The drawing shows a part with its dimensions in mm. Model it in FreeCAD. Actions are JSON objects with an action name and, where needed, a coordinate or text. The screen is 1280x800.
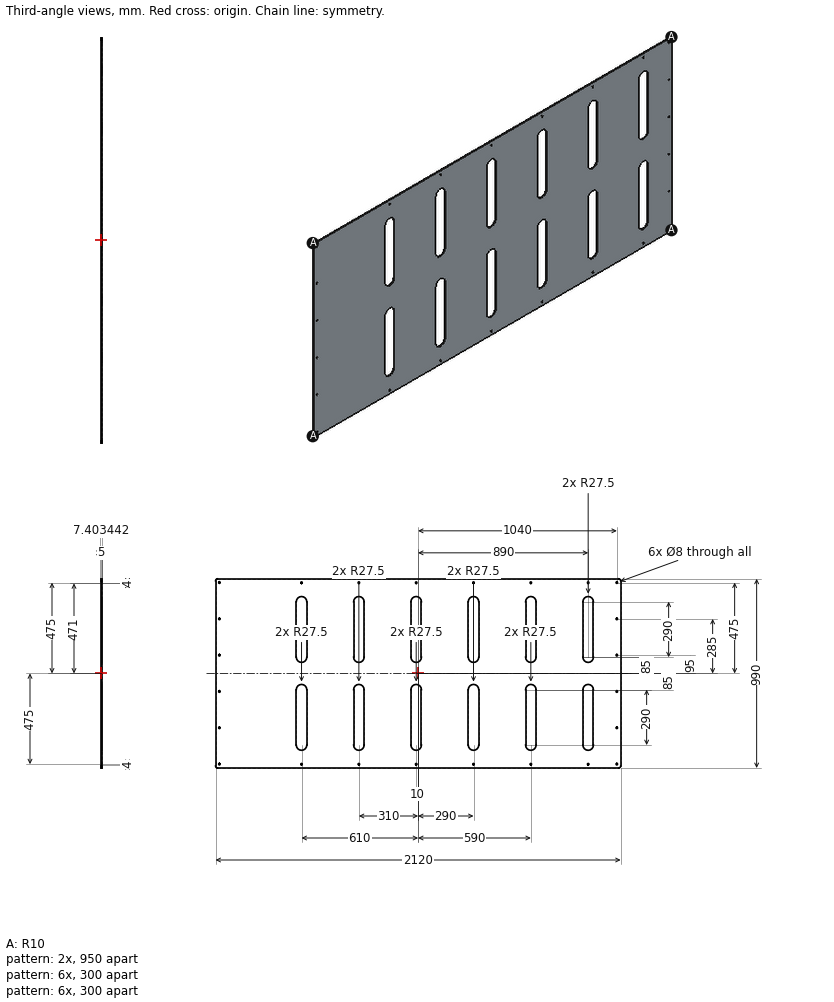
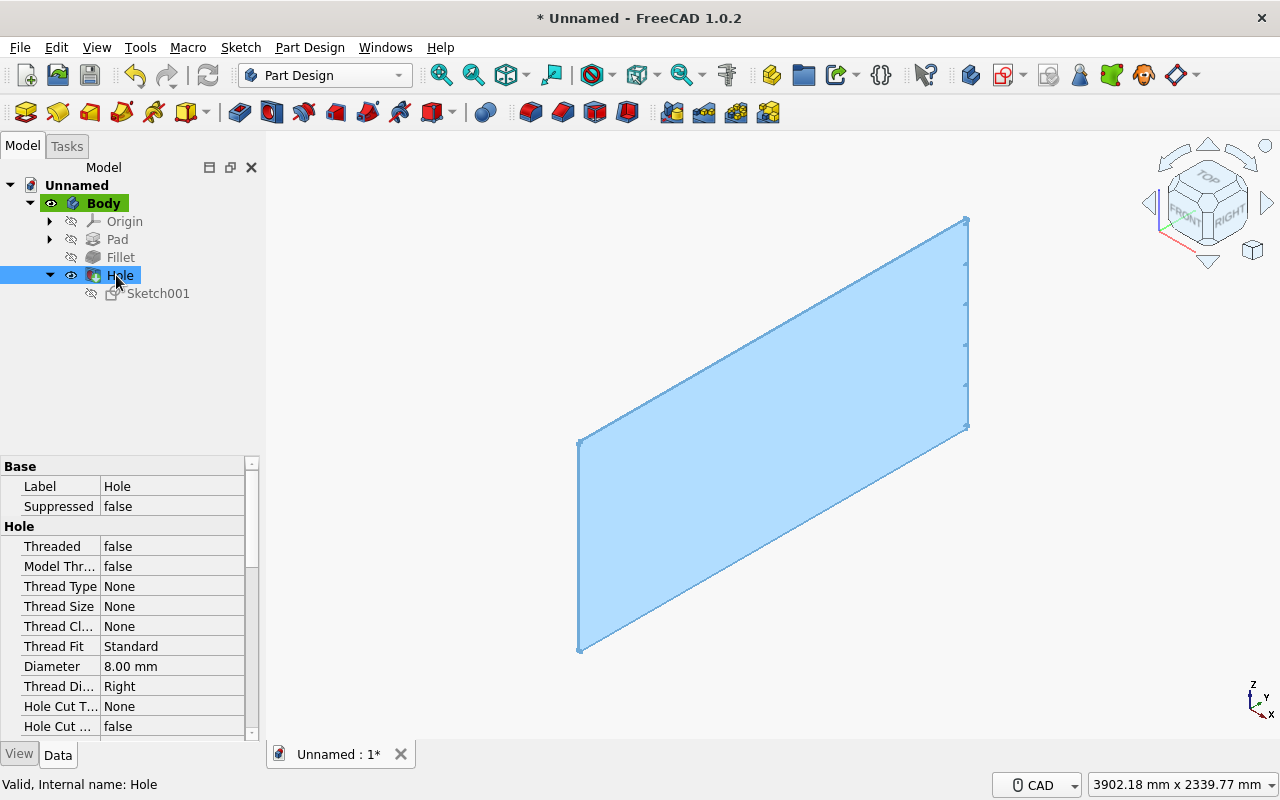
{"action": "left_click", "coordinate": [672, 112]}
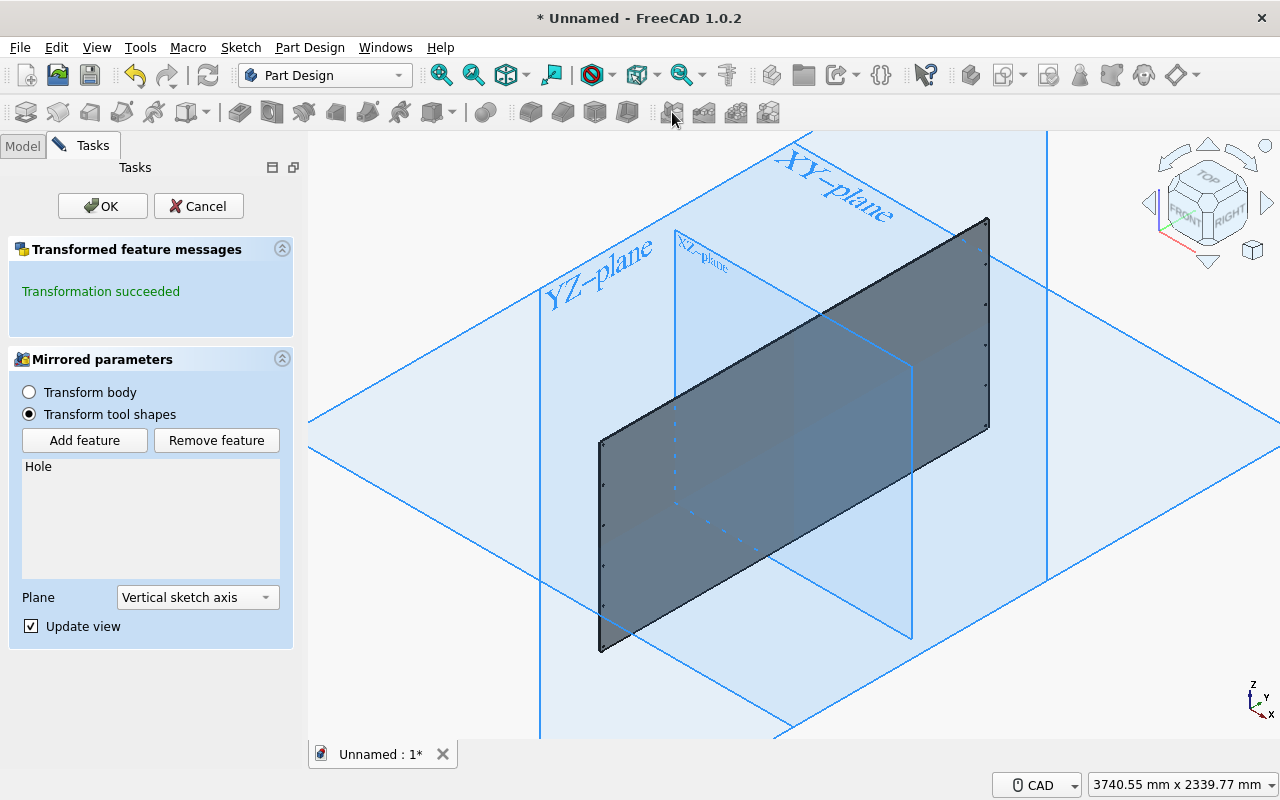
{"action": "left_click", "coordinate": [198, 598]}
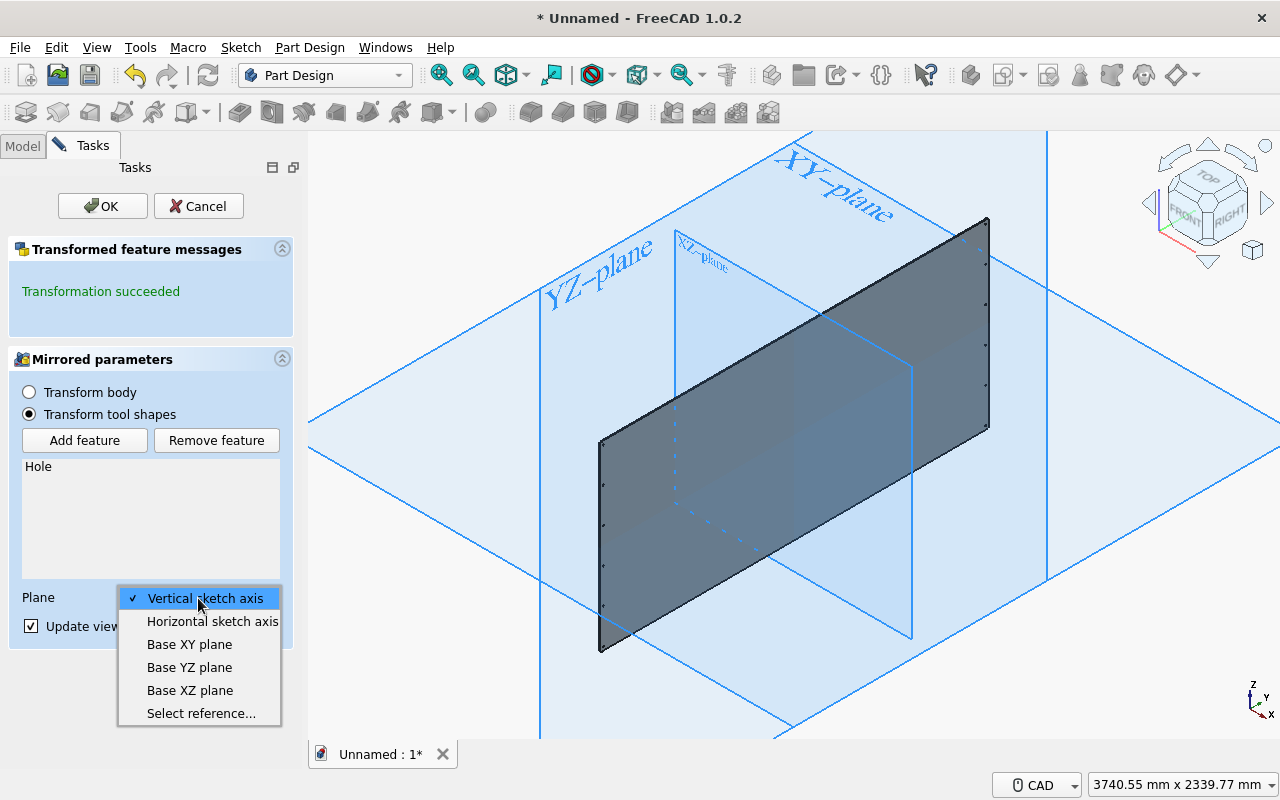
{"action": "left_click", "coordinate": [198, 690]}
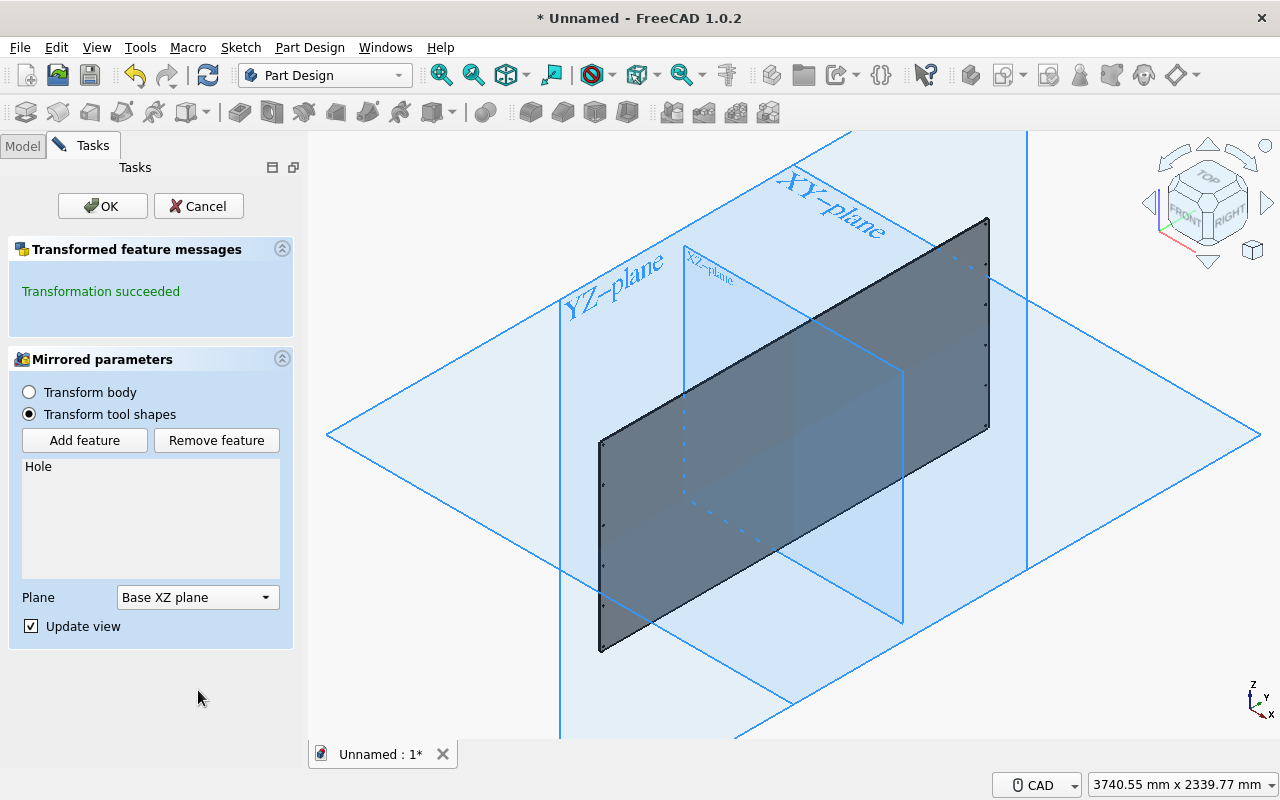
{"action": "left_click", "coordinate": [103, 206]}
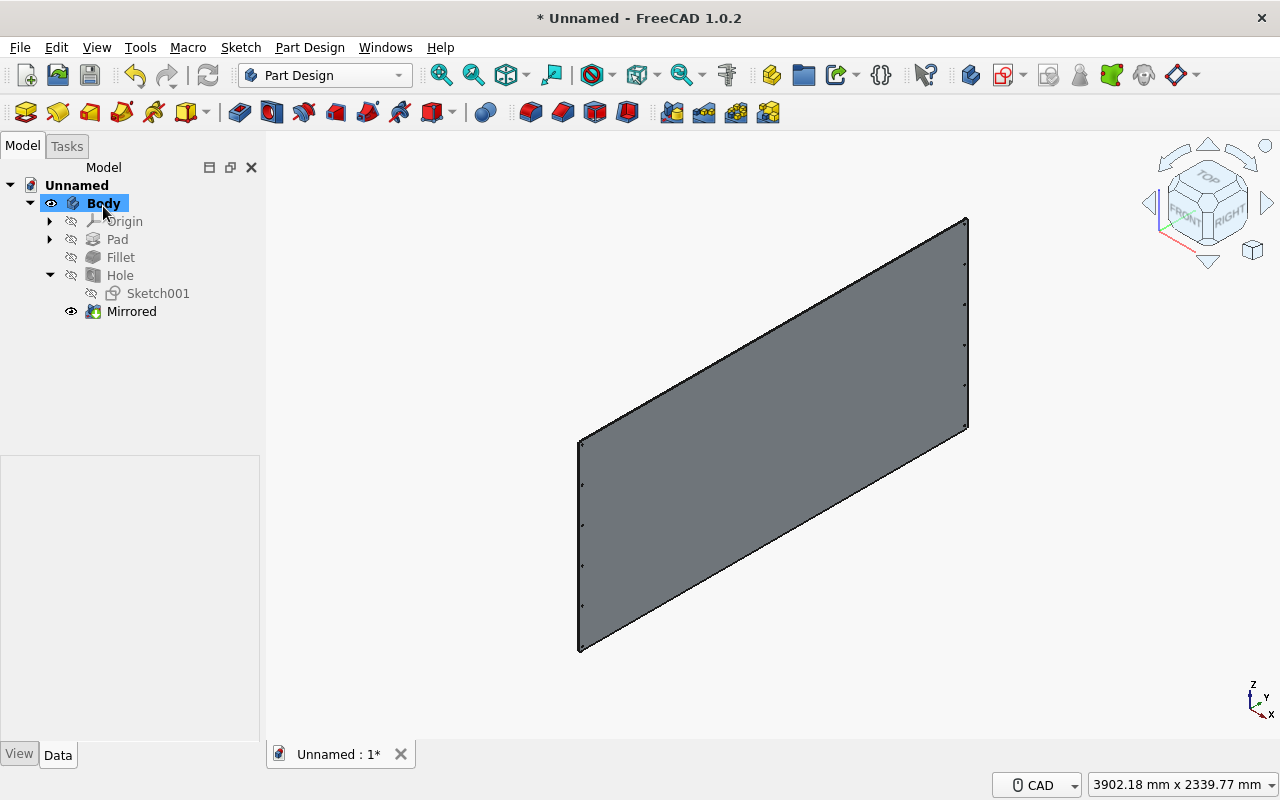
{"action": "left_click", "coordinate": [50, 221]}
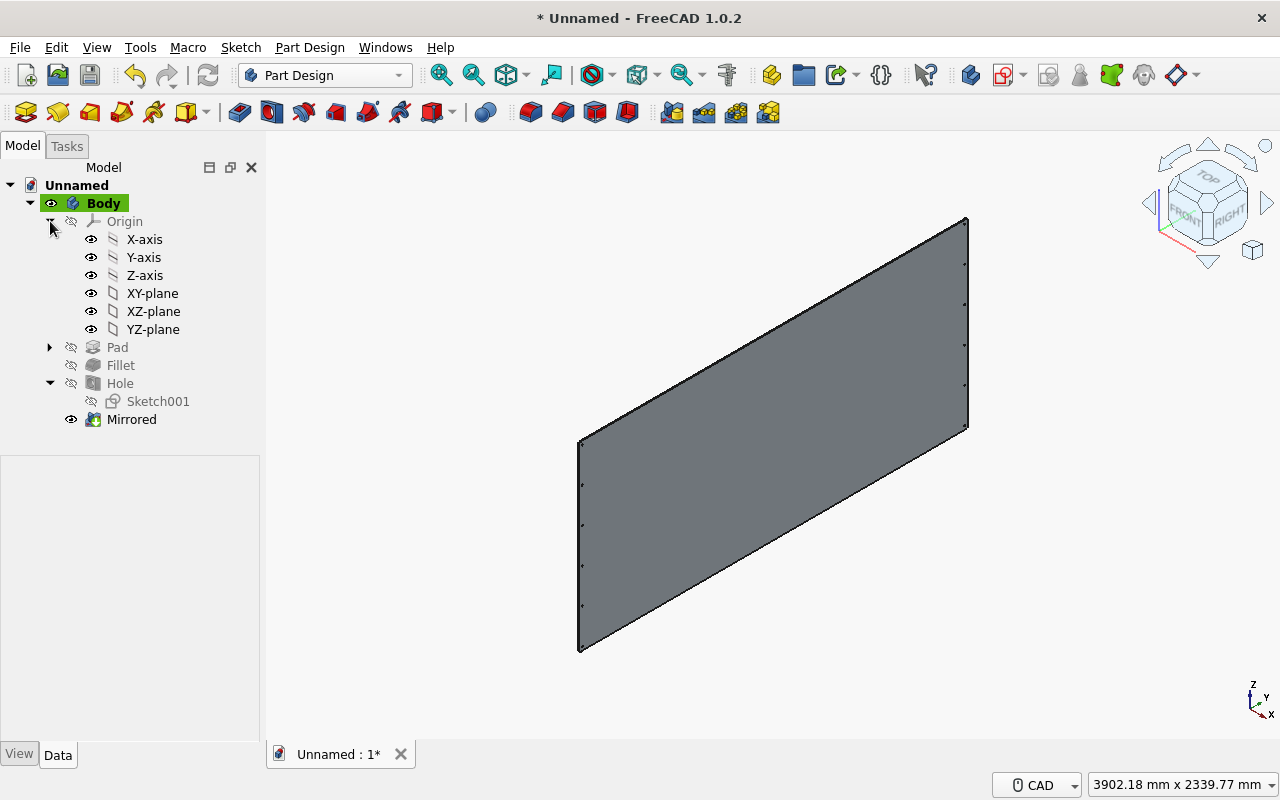
{"action": "left_click", "coordinate": [136, 311]}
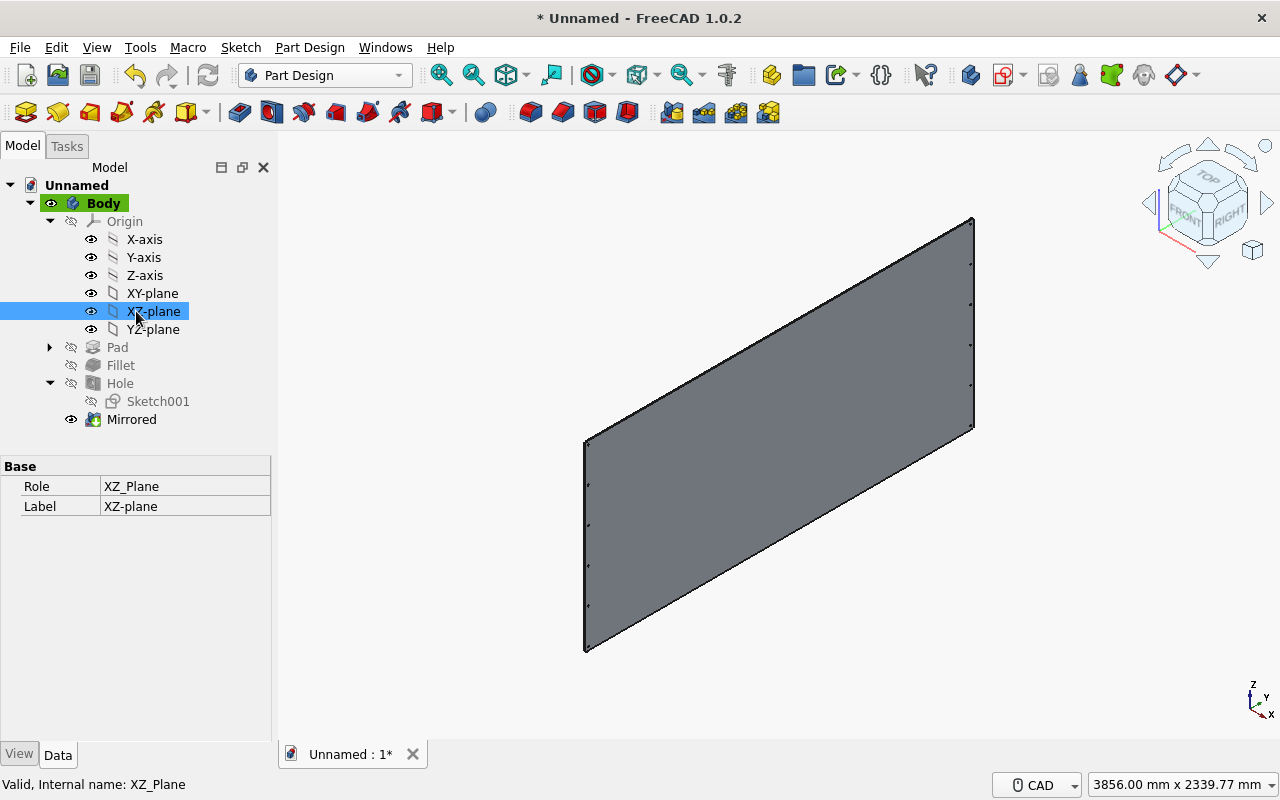
{"action": "left_click", "coordinate": [1176, 76]}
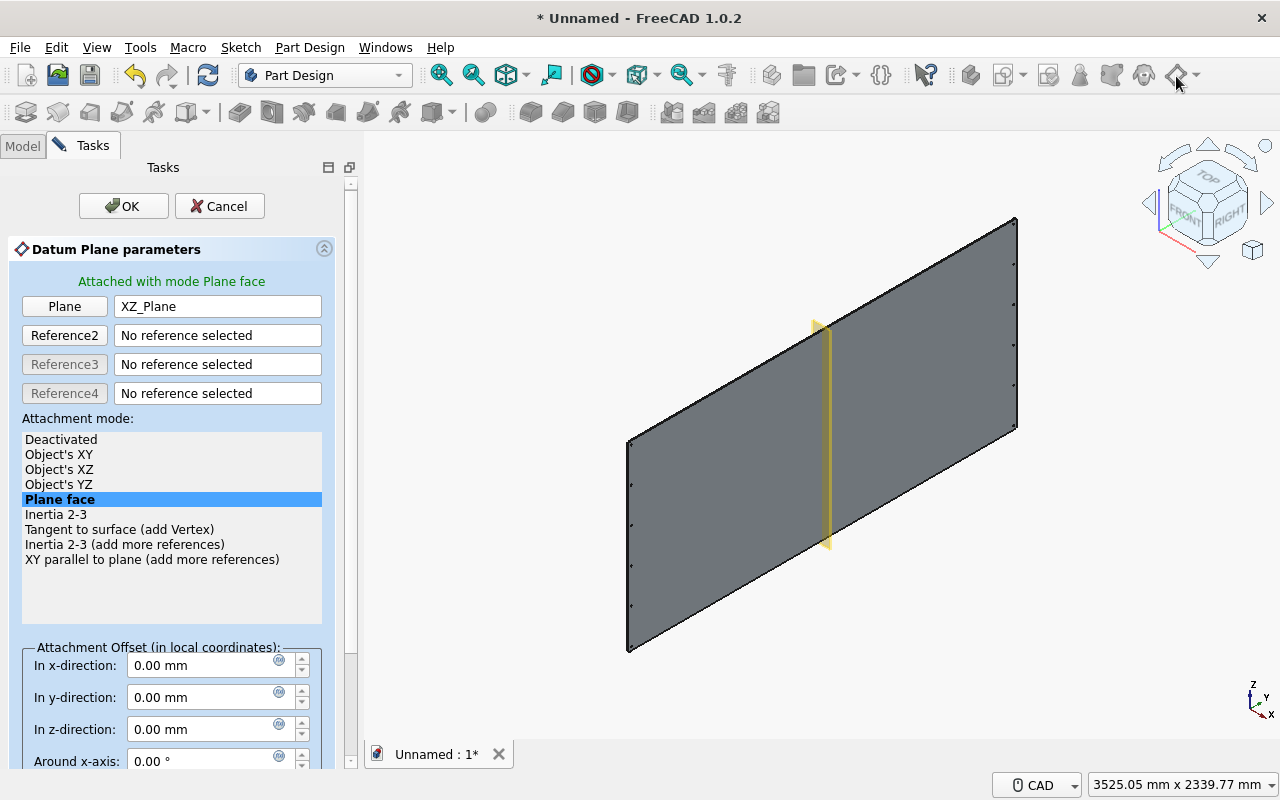
{"action": "triple_click", "coordinate": [210, 729]}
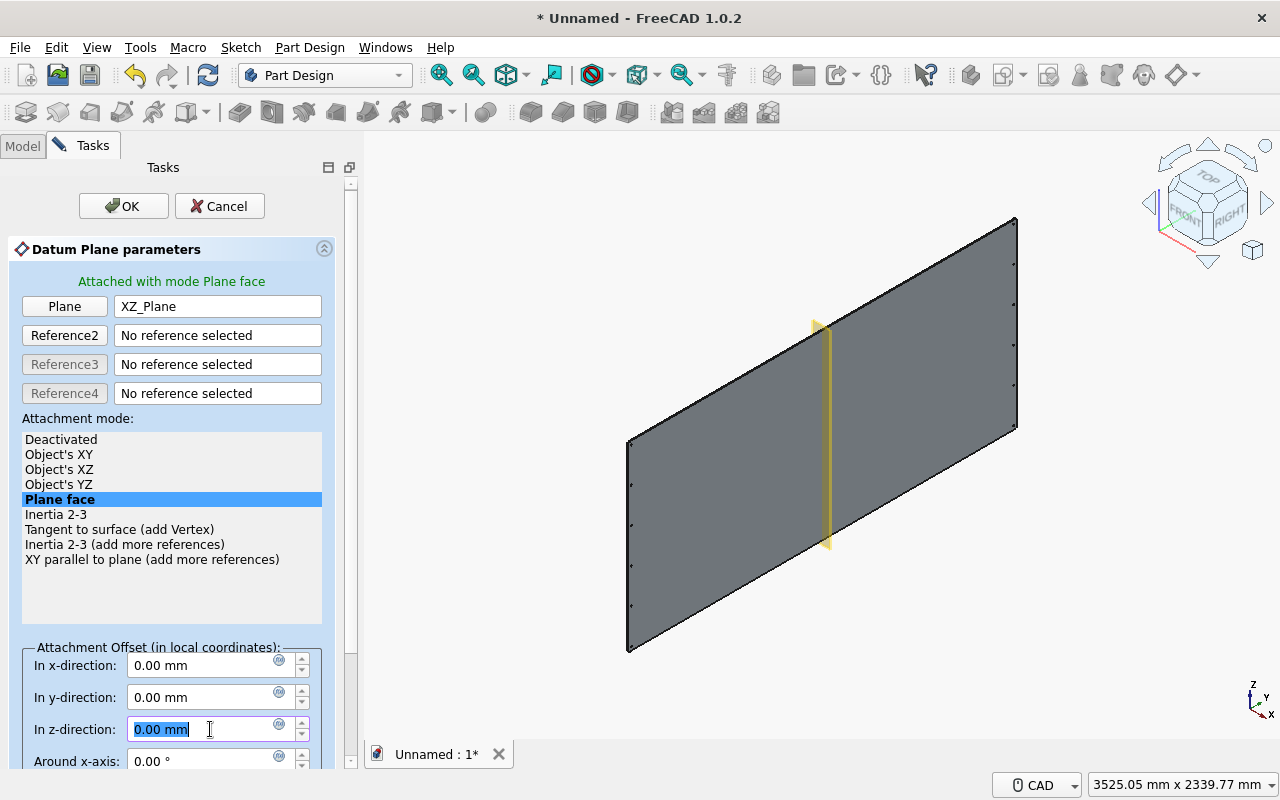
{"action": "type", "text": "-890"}
{"action": "key", "text": "Tab"}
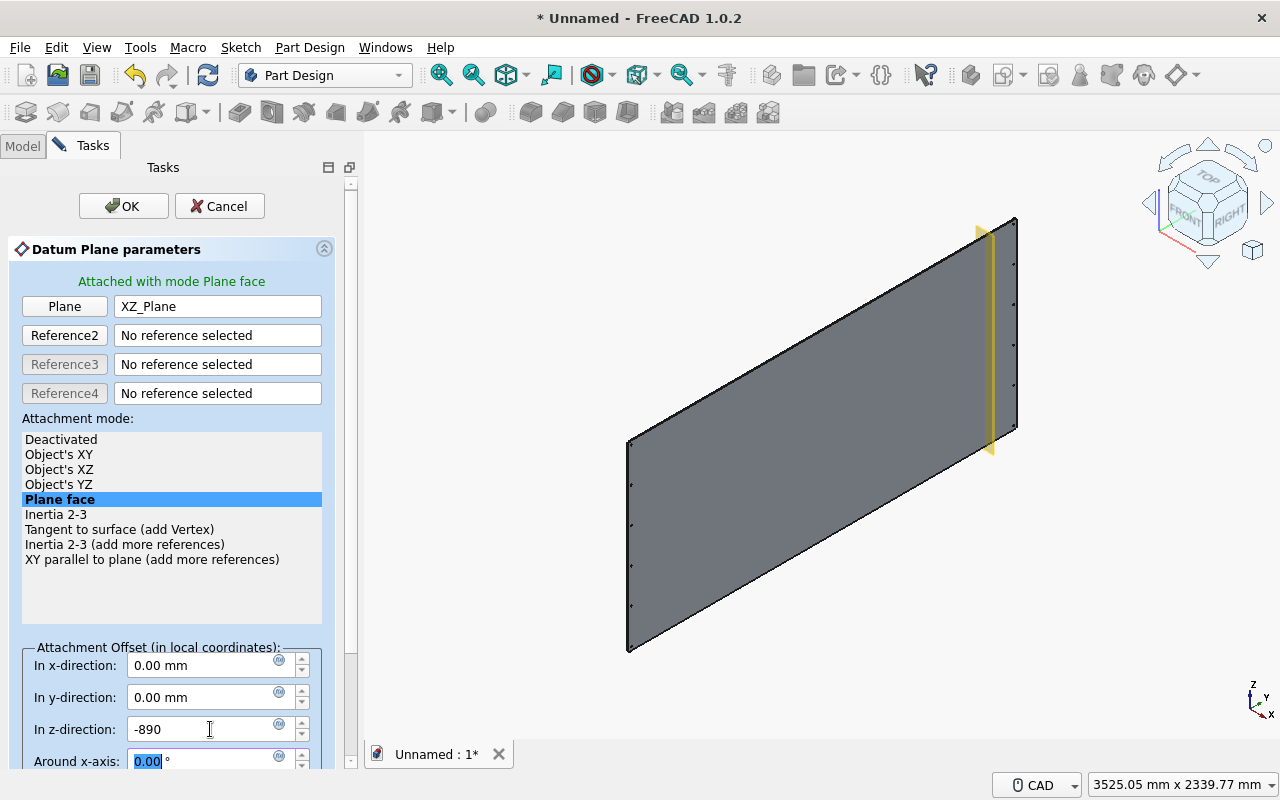
{"action": "left_click", "coordinate": [124, 206]}